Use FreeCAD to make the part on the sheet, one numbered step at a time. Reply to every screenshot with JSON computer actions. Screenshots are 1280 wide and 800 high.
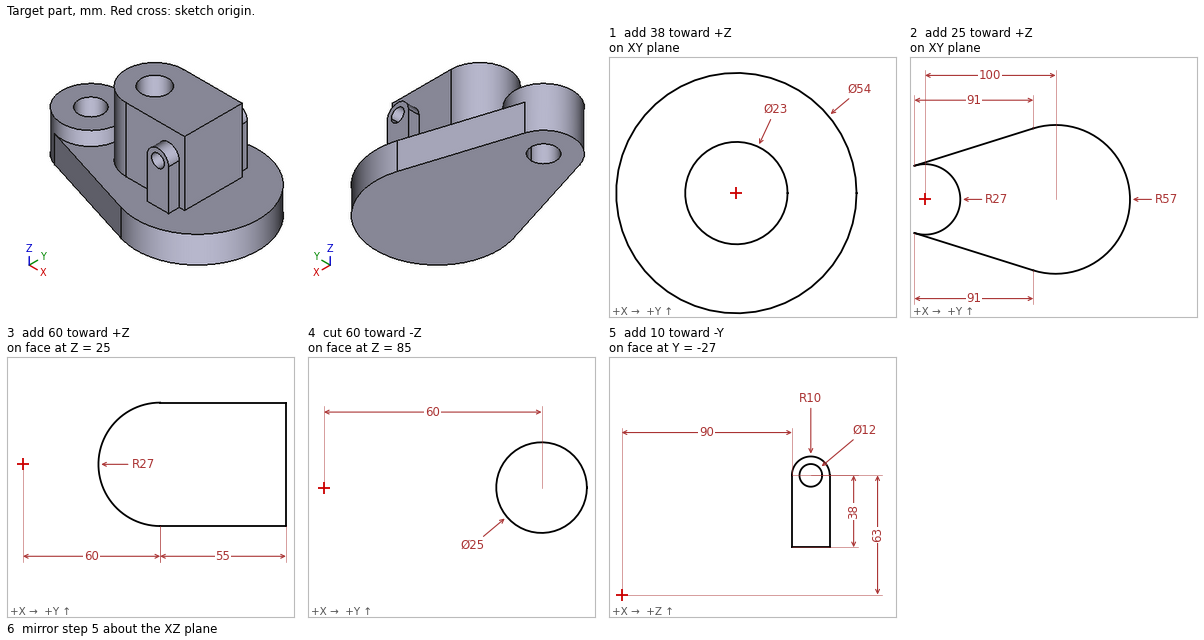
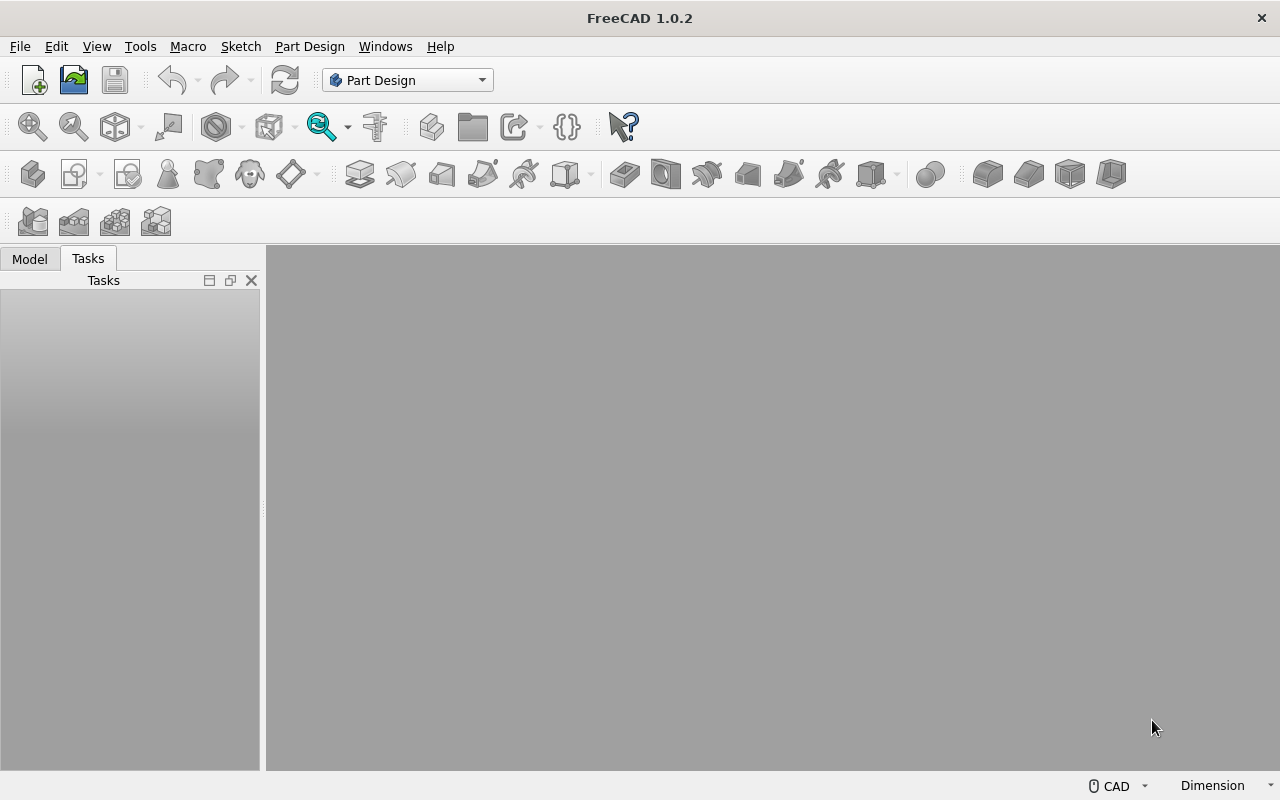
{"action": "key", "text": "ctrl+n"}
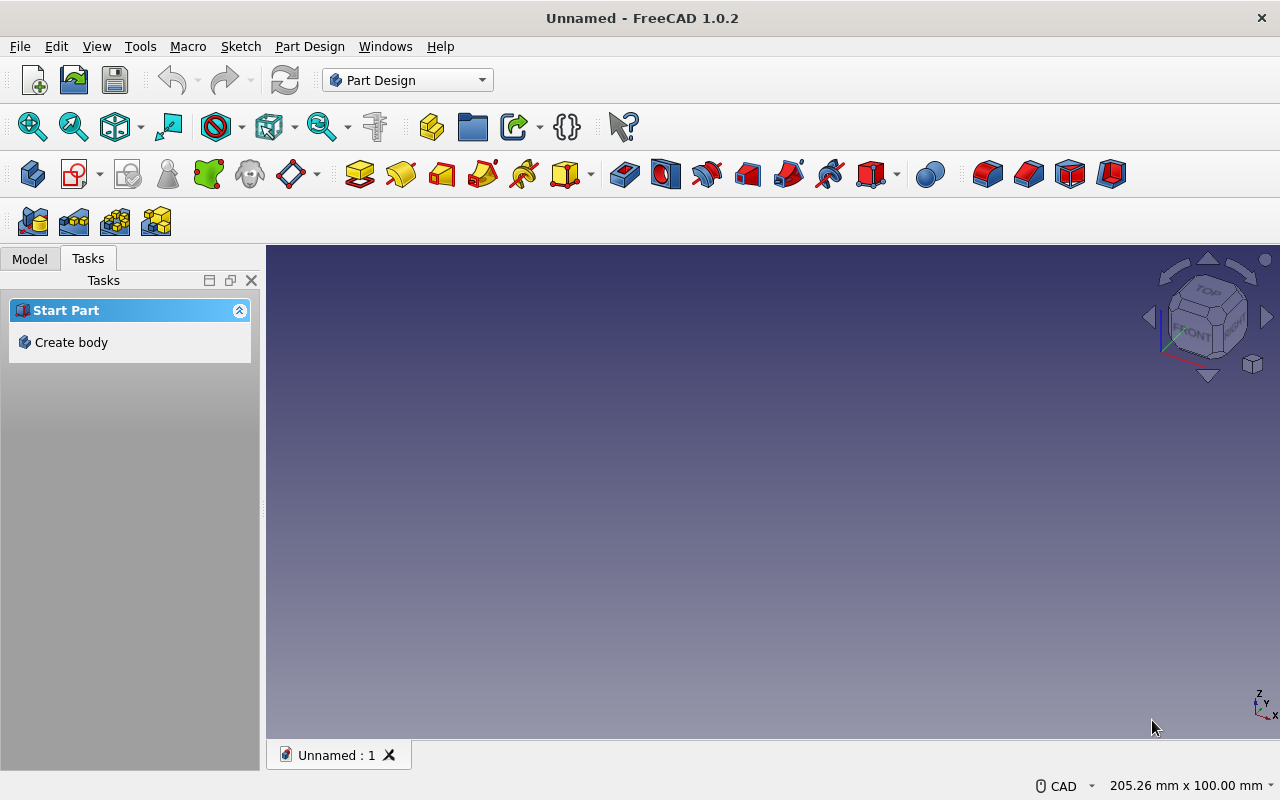
{"action": "left_click", "coordinate": [74, 174]}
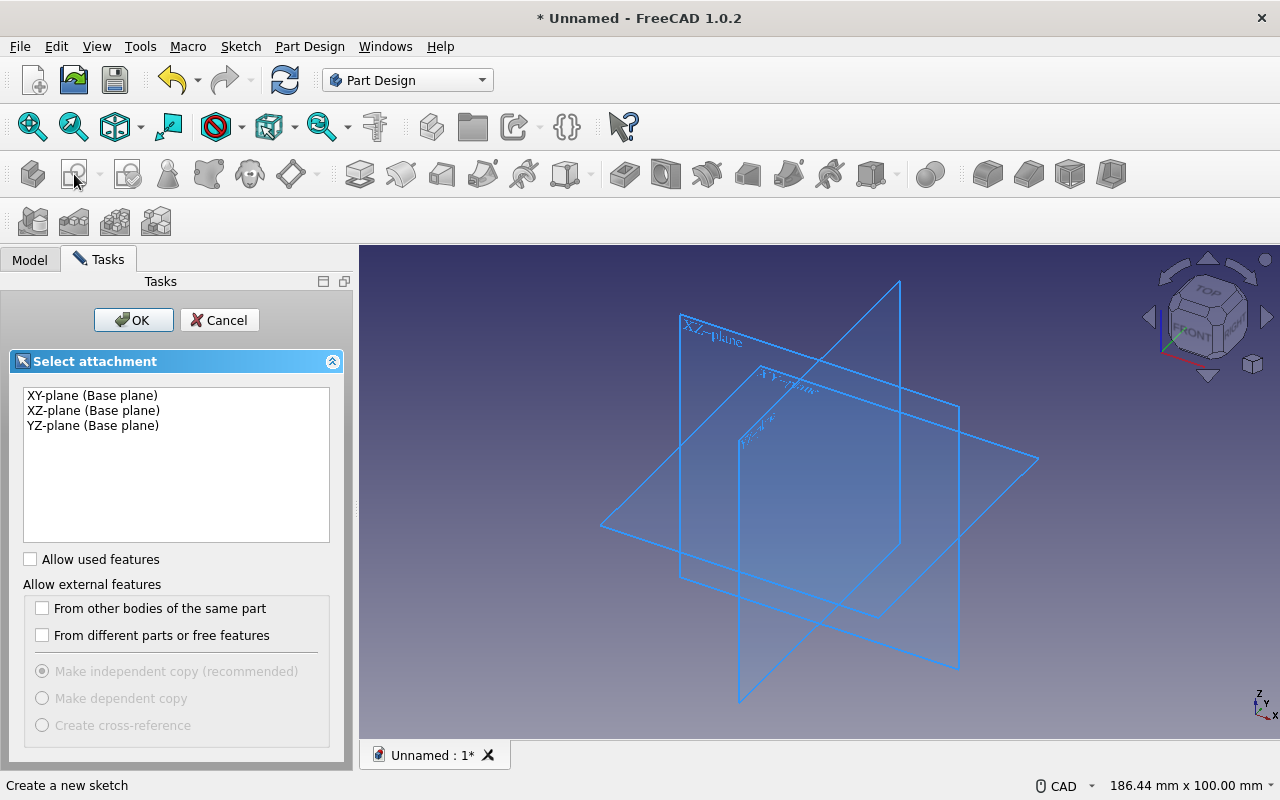
{"action": "left_click", "coordinate": [84, 396]}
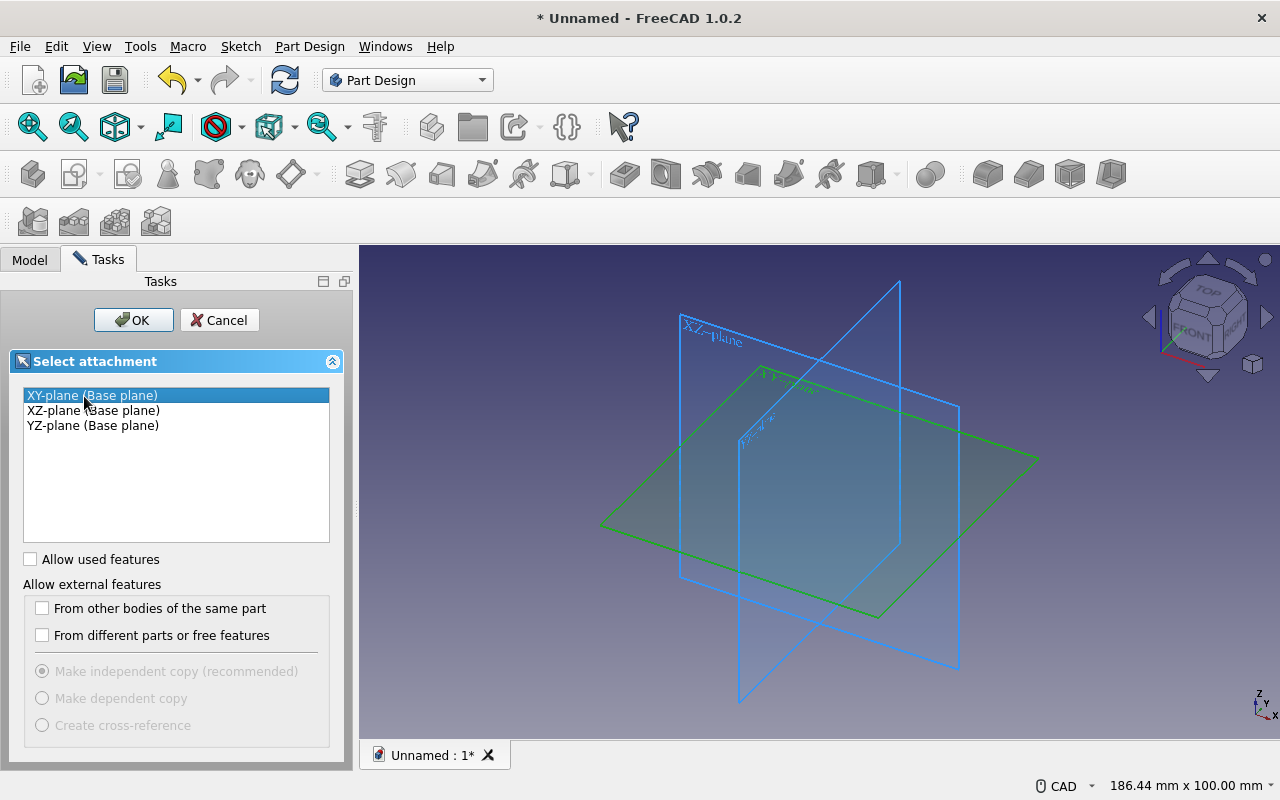
{"action": "left_click", "coordinate": [134, 320]}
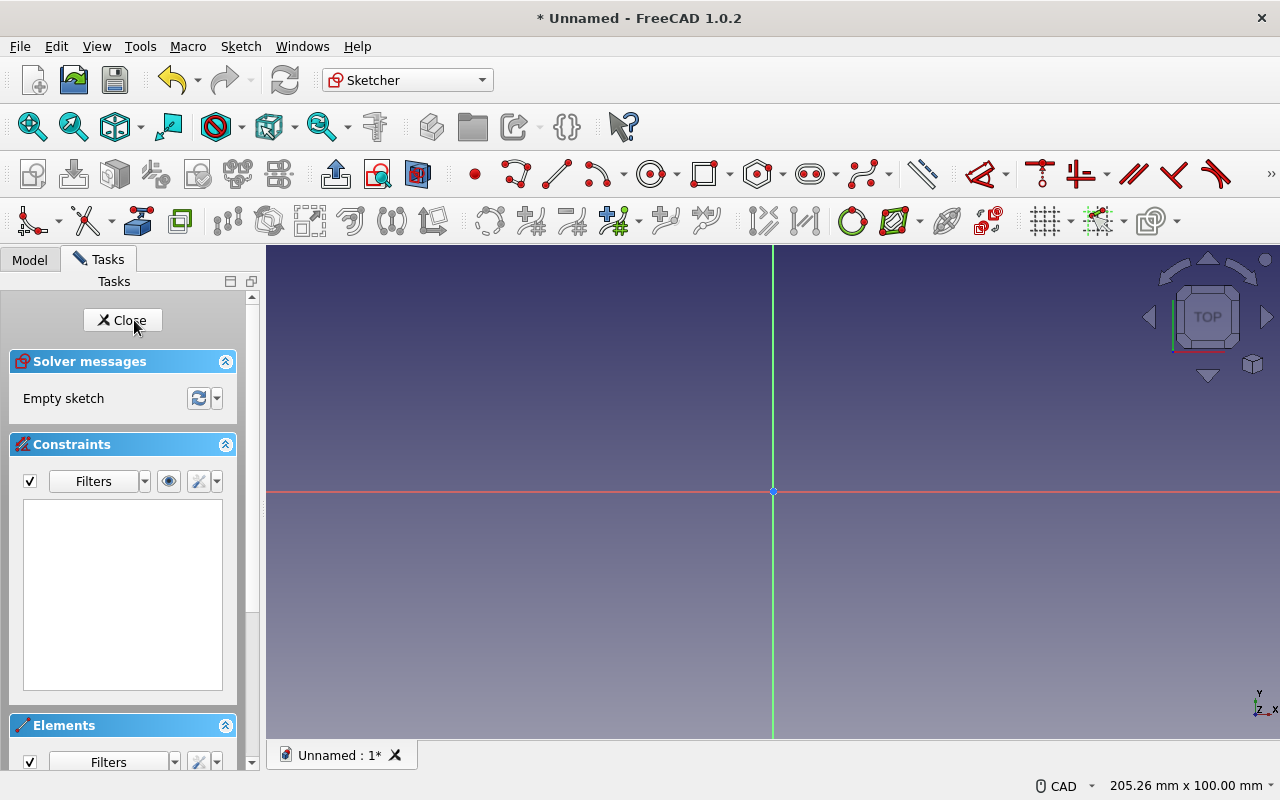
{"action": "left_click", "coordinate": [650, 174]}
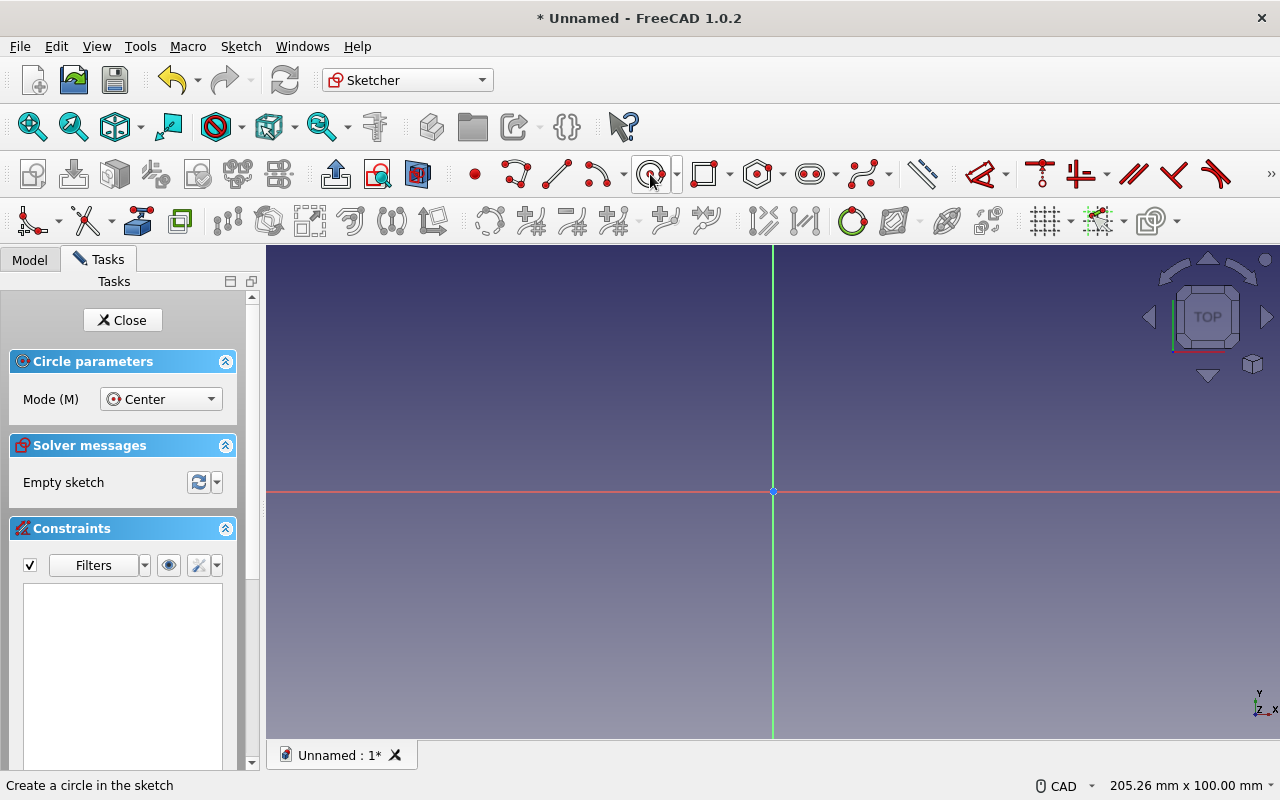
{"action": "left_click", "coordinate": [773, 492]}
{"action": "mouse_move", "coordinate": [867, 398]}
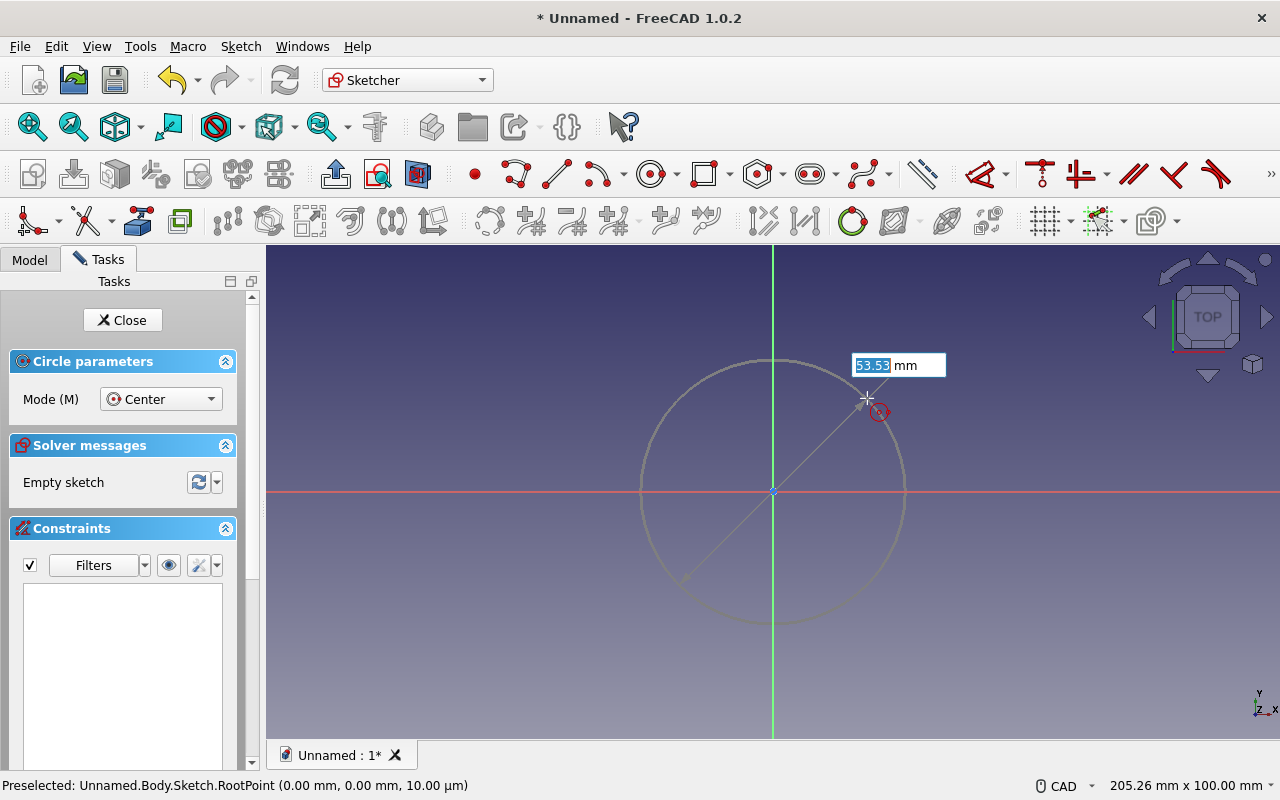
{"action": "type", "text": "54"}
{"action": "key", "text": "Return"}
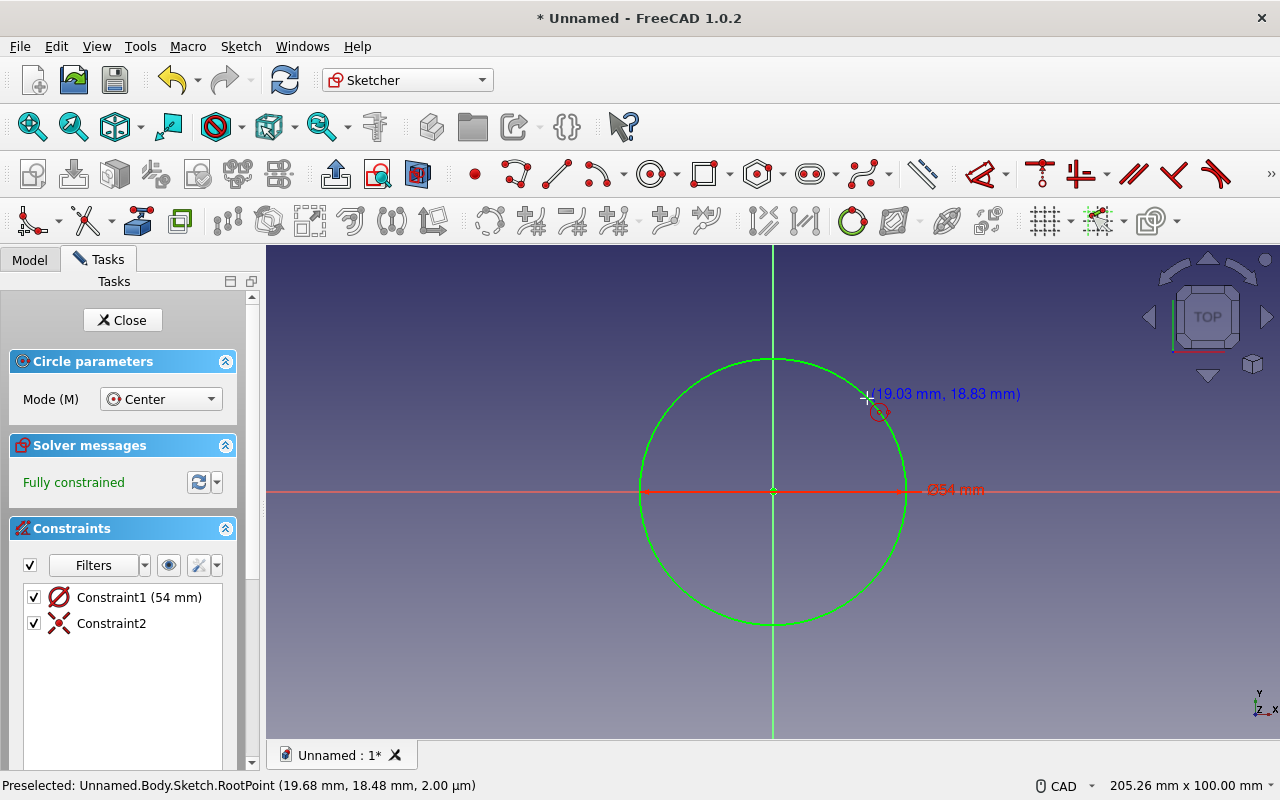
{"action": "left_click", "coordinate": [773, 492]}
{"action": "mouse_move", "coordinate": [813, 452]}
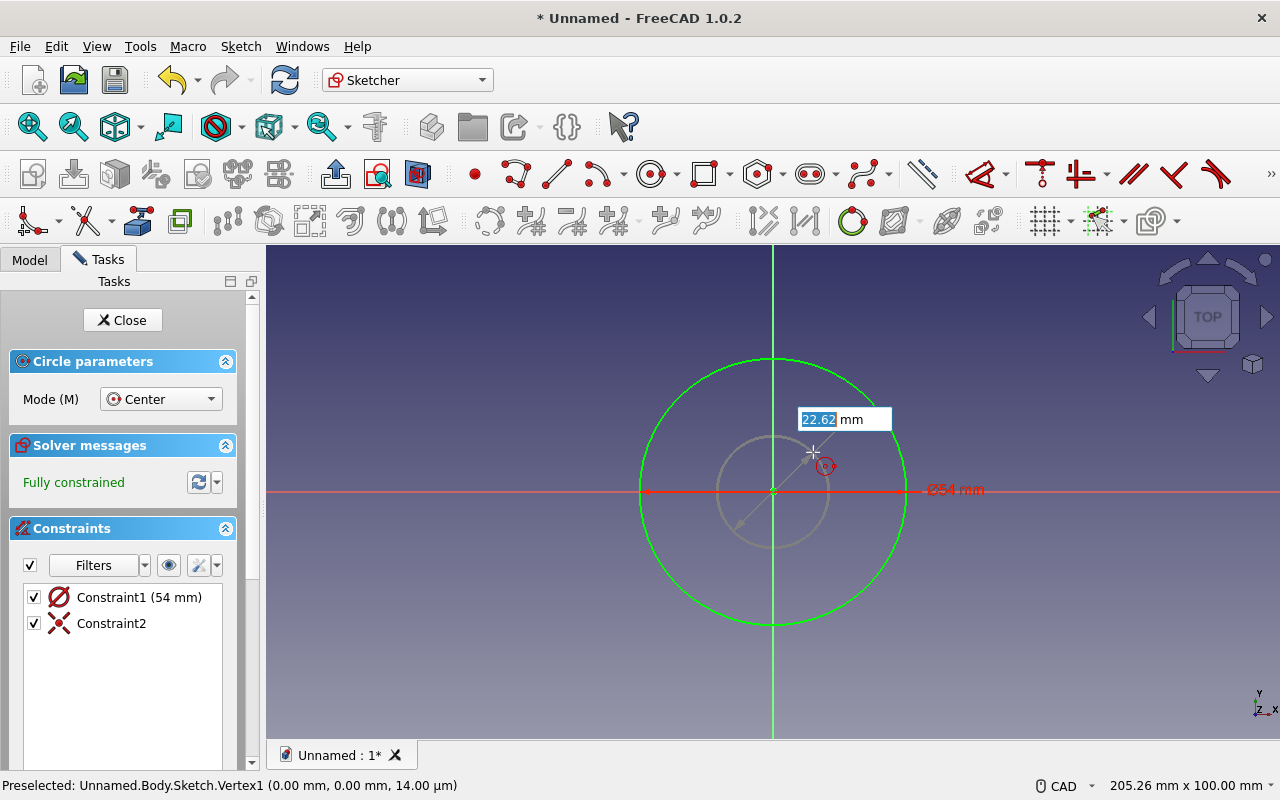
{"action": "type", "text": "23"}
{"action": "key", "text": "Return"}
{"action": "key", "text": "Escape"}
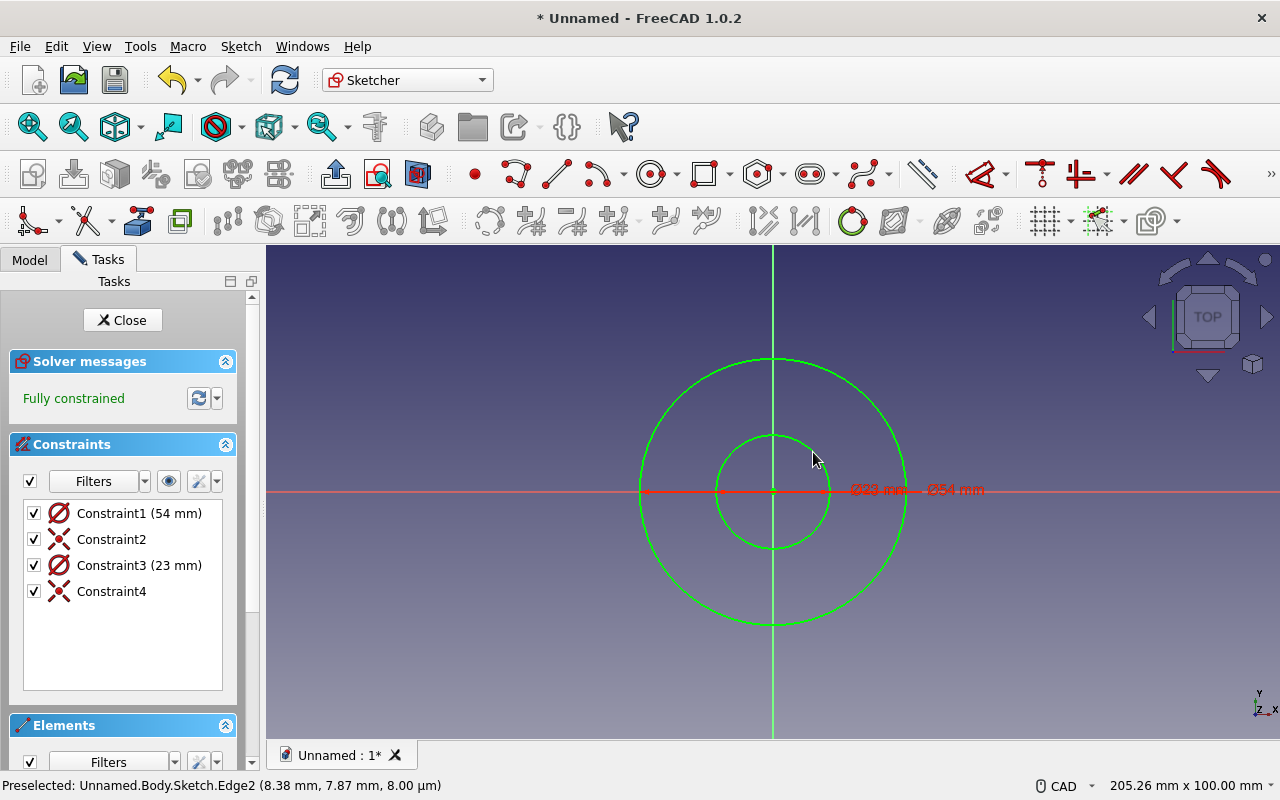
{"action": "left_click", "coordinate": [123, 320]}